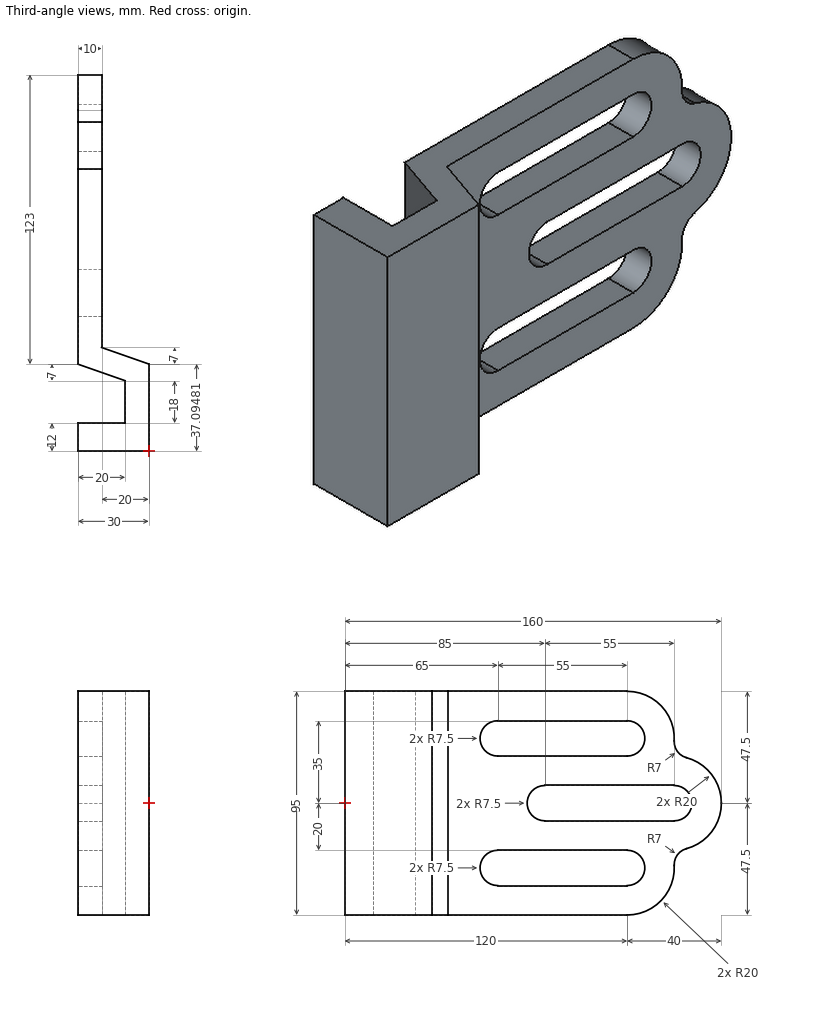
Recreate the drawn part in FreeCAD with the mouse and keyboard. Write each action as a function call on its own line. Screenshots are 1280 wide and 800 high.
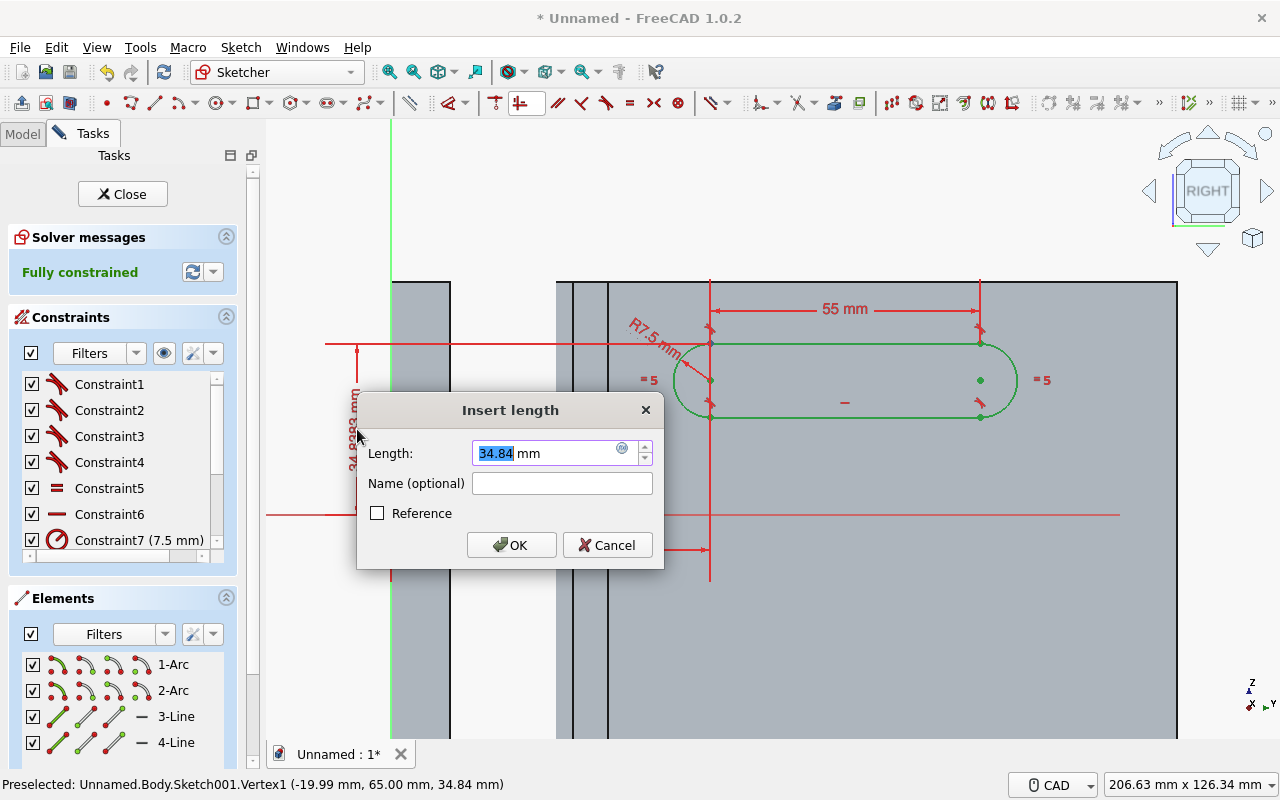
text(35)
key(Return)
key(Escape)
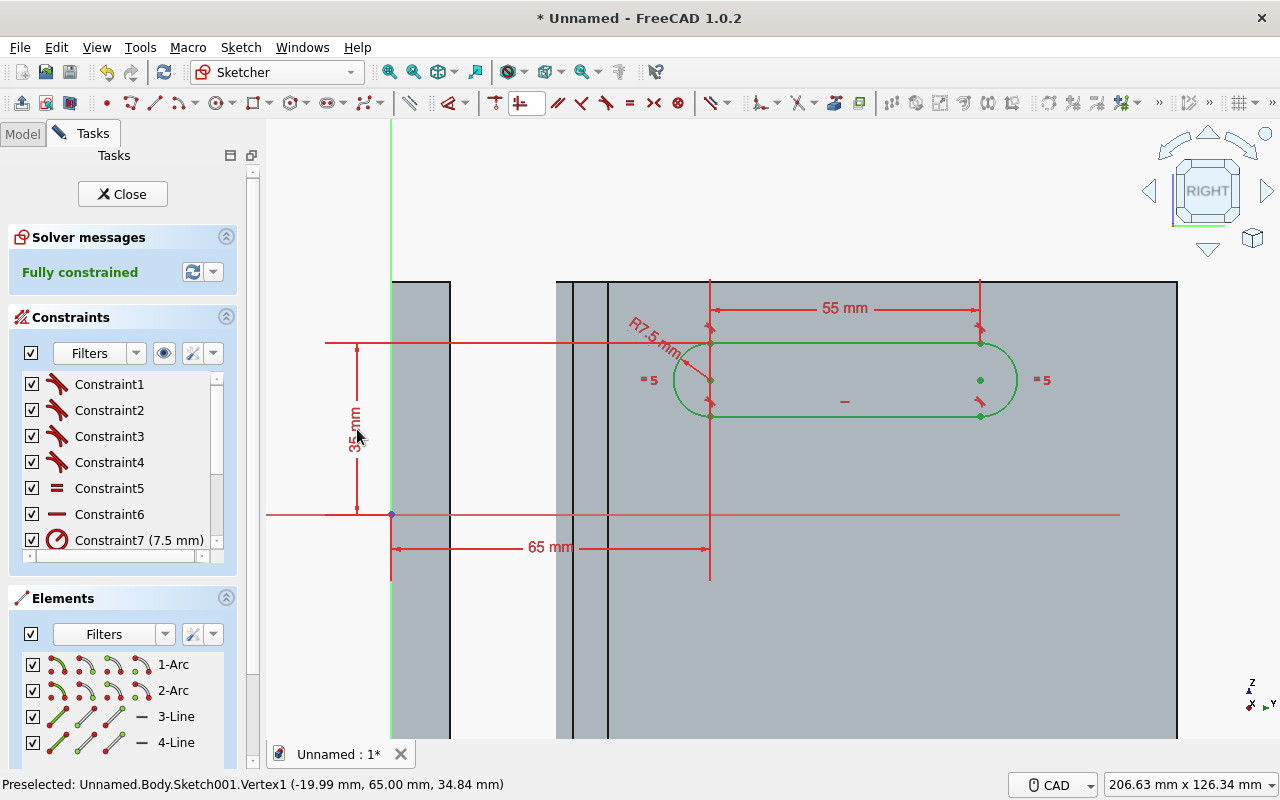
click(123, 194)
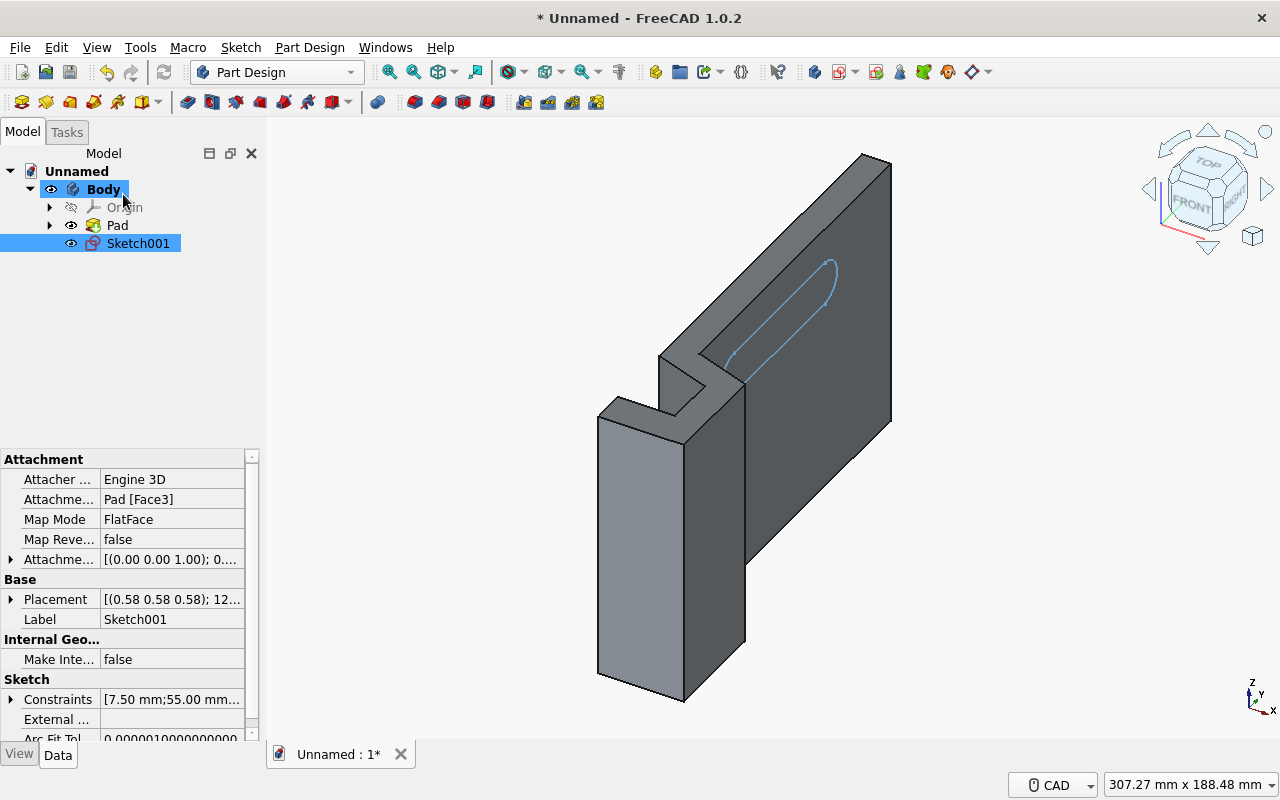
click(188, 102)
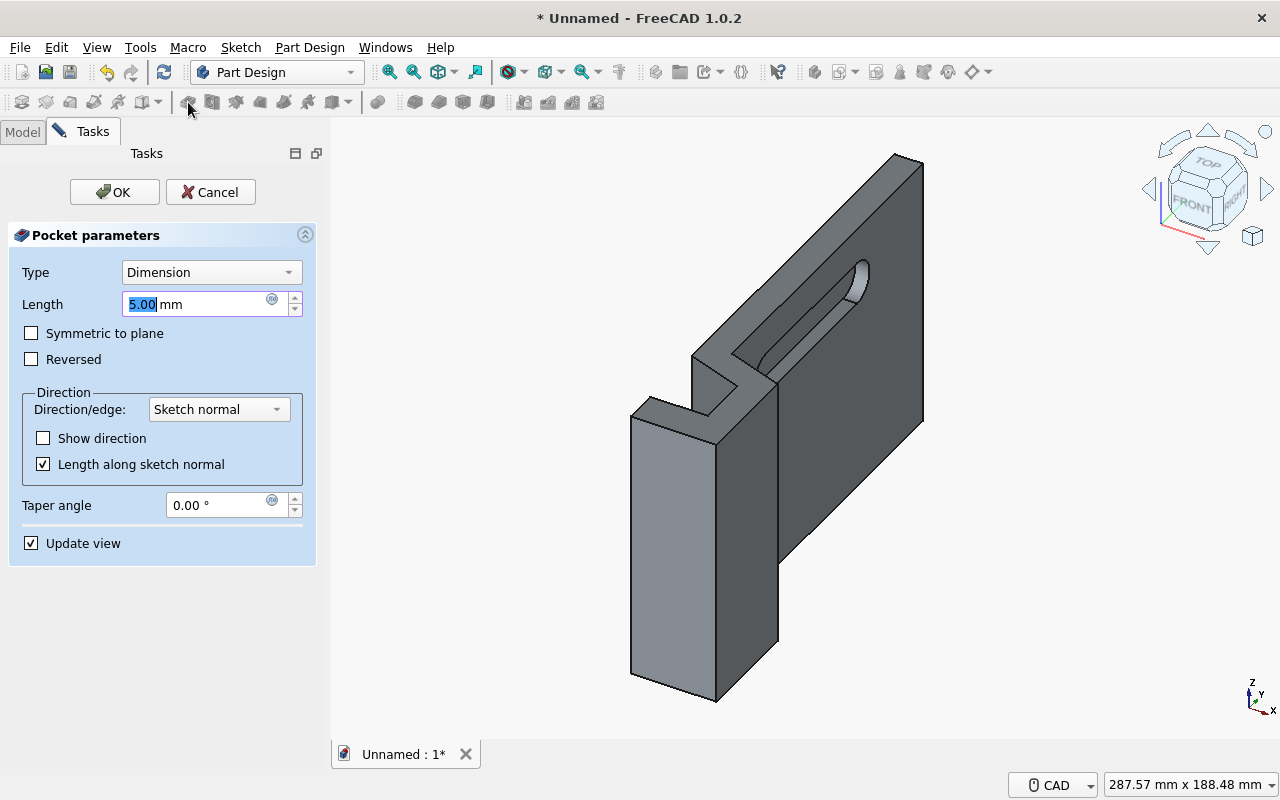
click(212, 272)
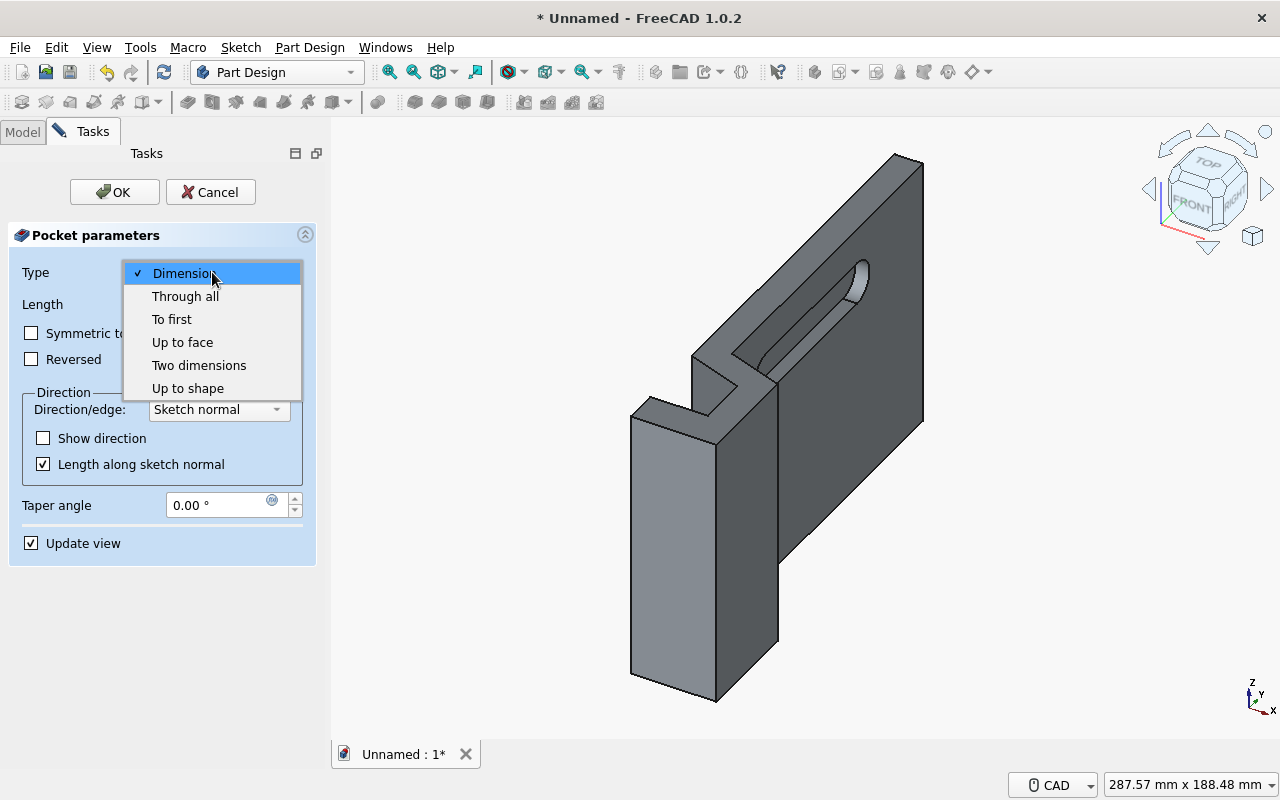
click(212, 320)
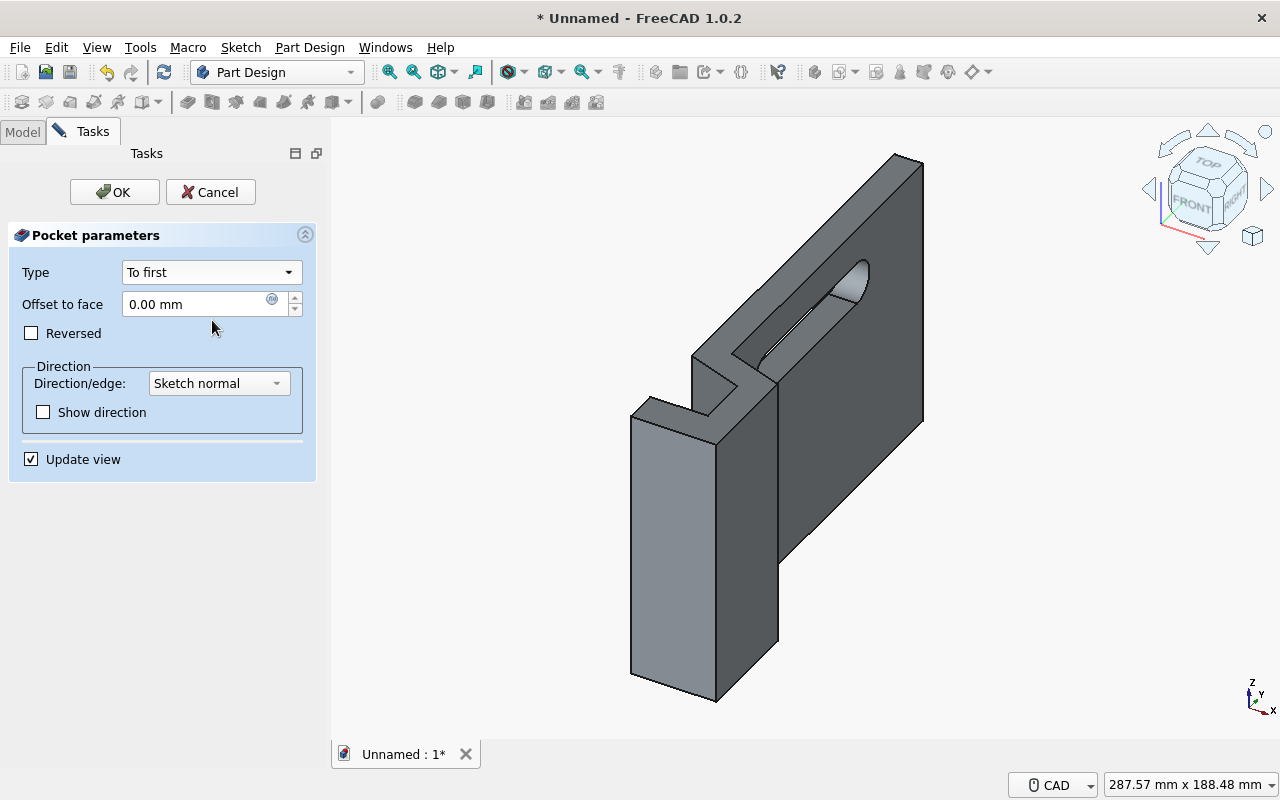
click(115, 192)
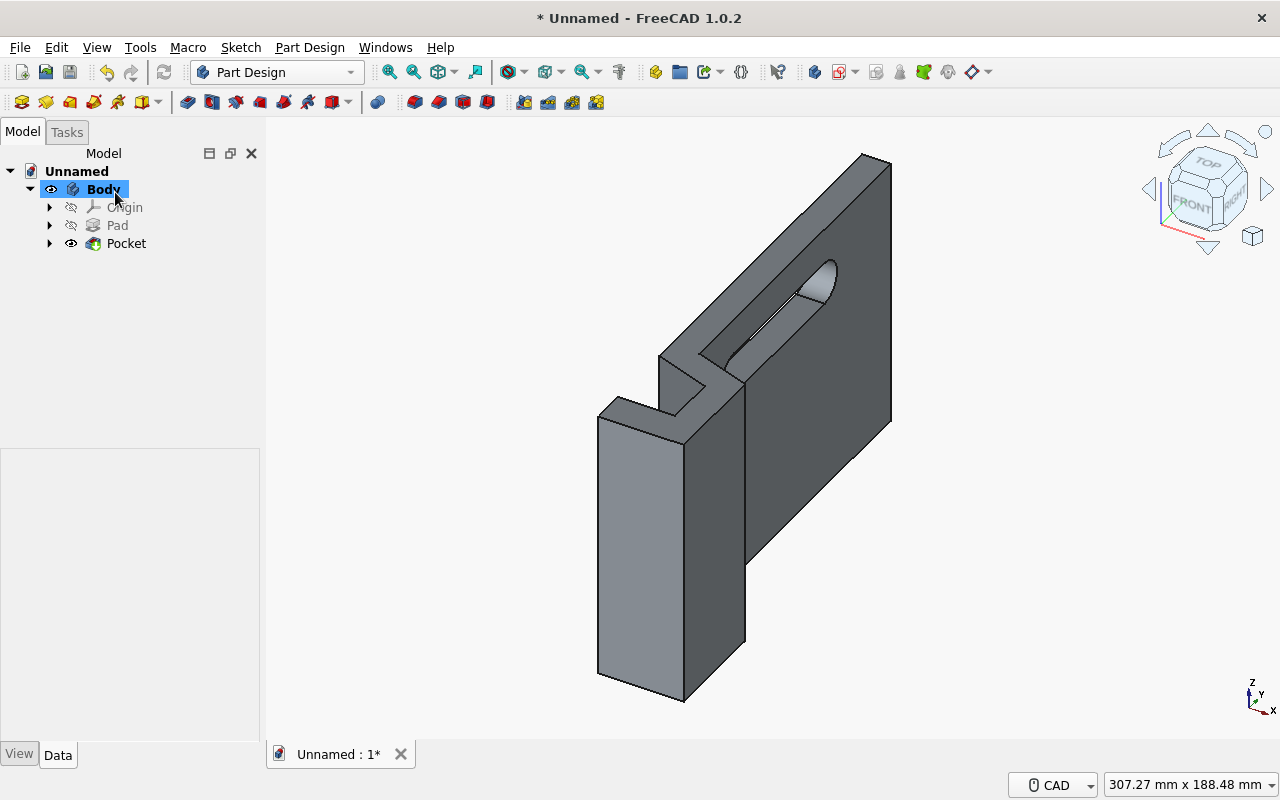
click(822, 396)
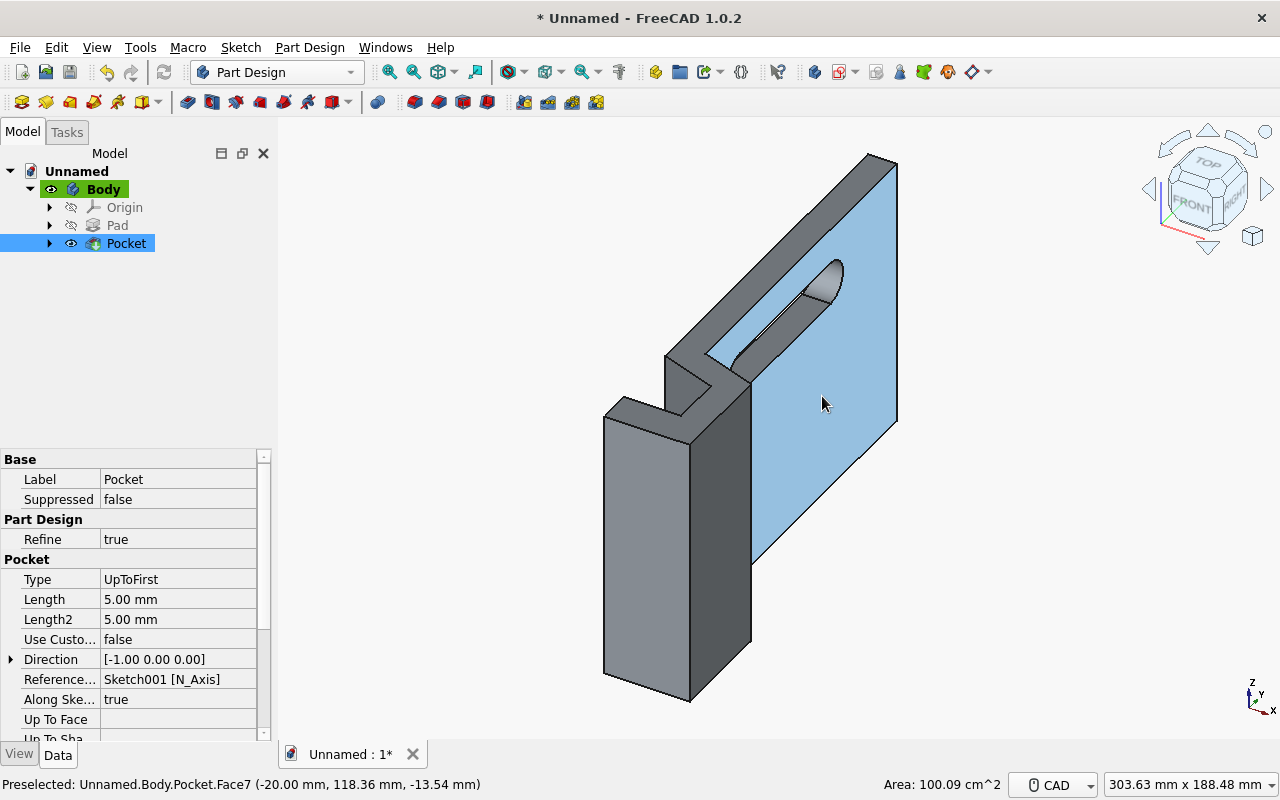
click(840, 72)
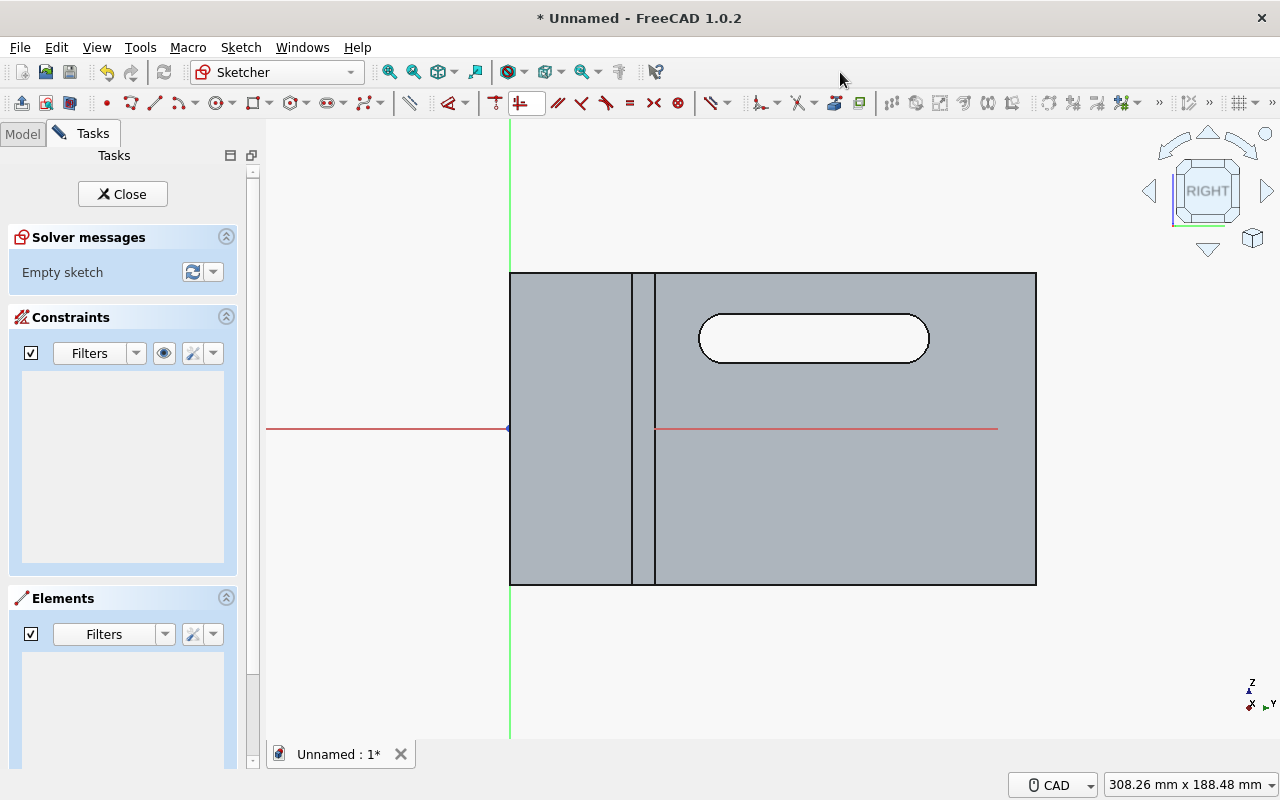
click(328, 104)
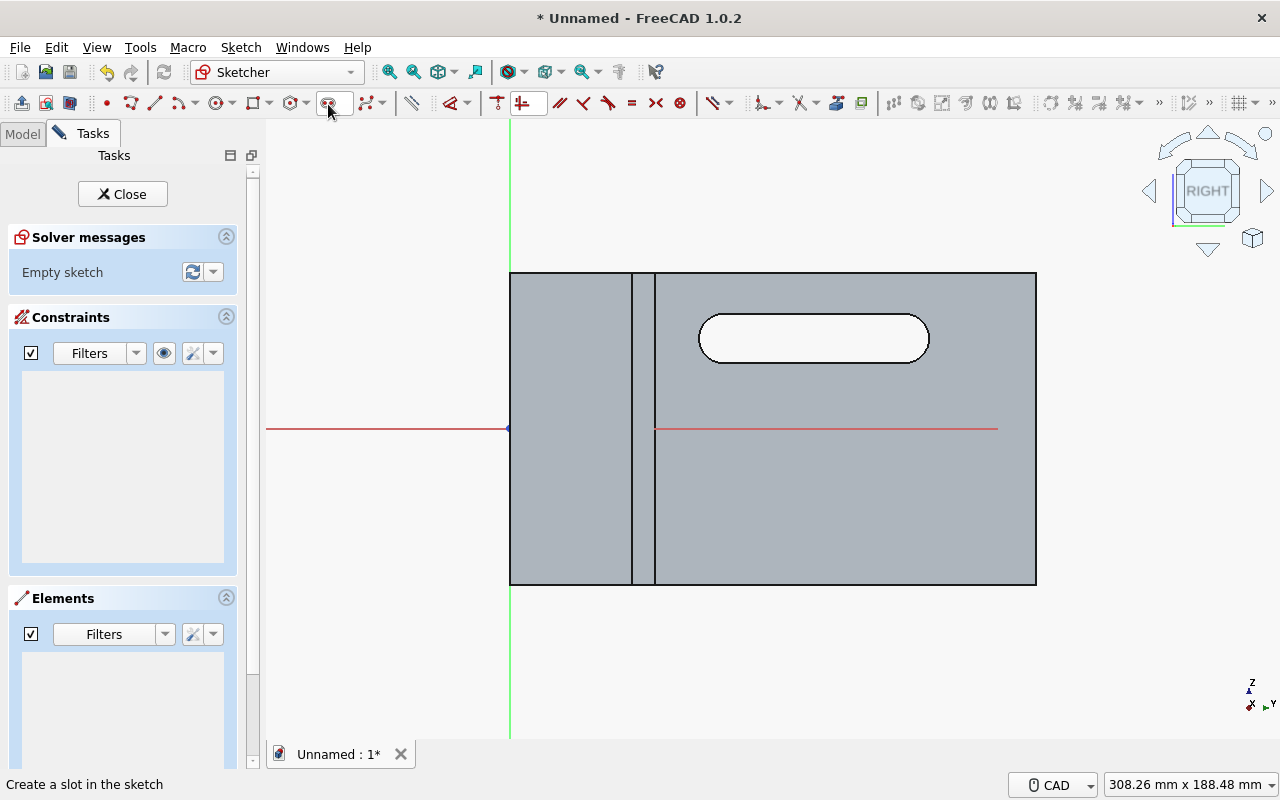
click(789, 429)